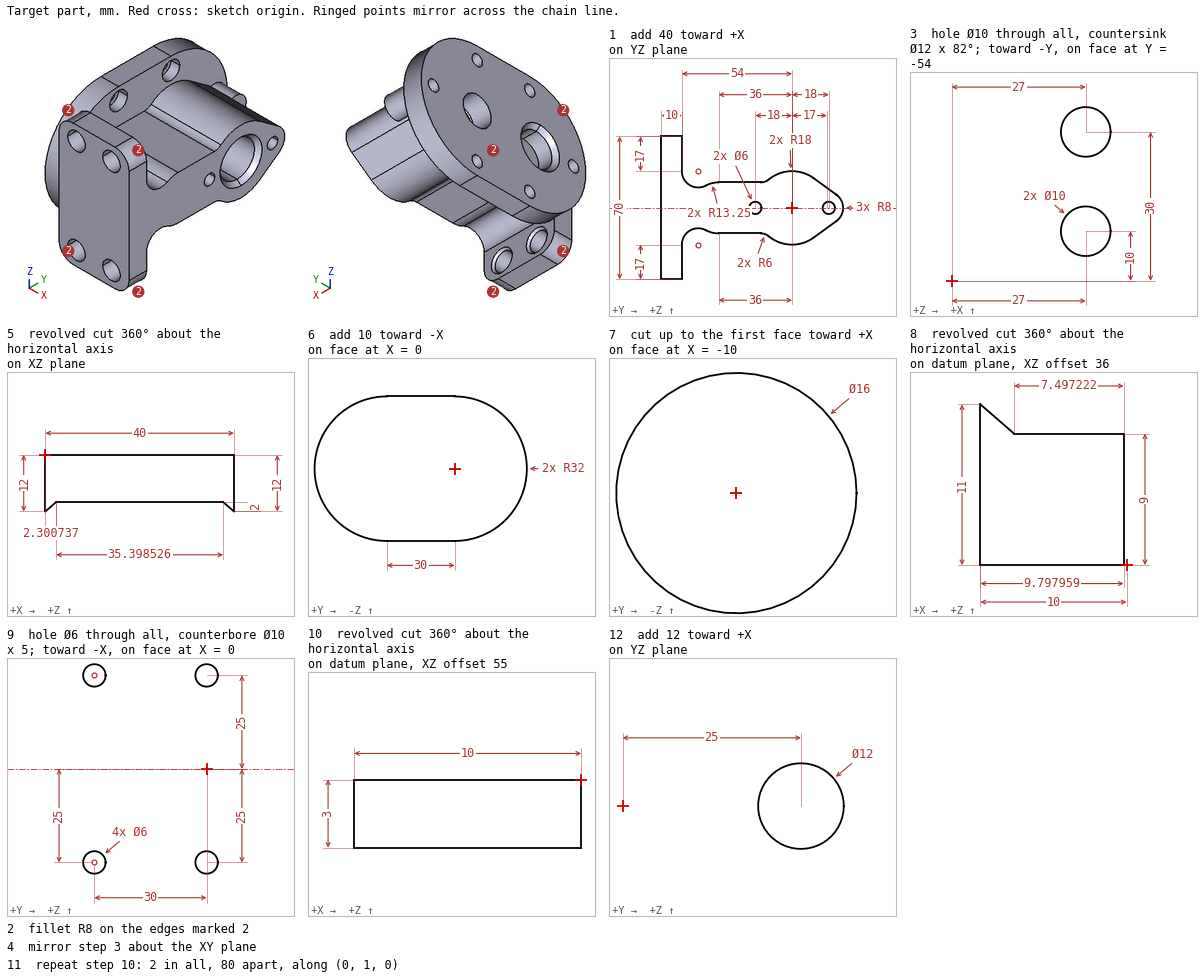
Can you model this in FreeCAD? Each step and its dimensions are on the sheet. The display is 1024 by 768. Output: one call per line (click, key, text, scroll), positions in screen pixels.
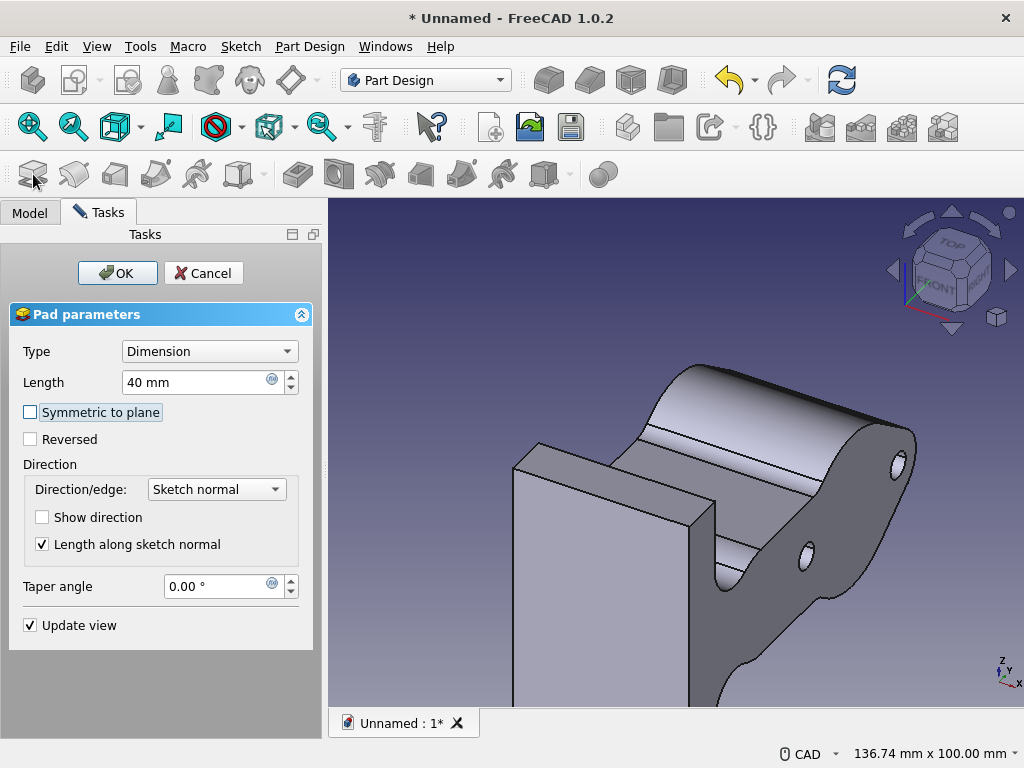
click(118, 273)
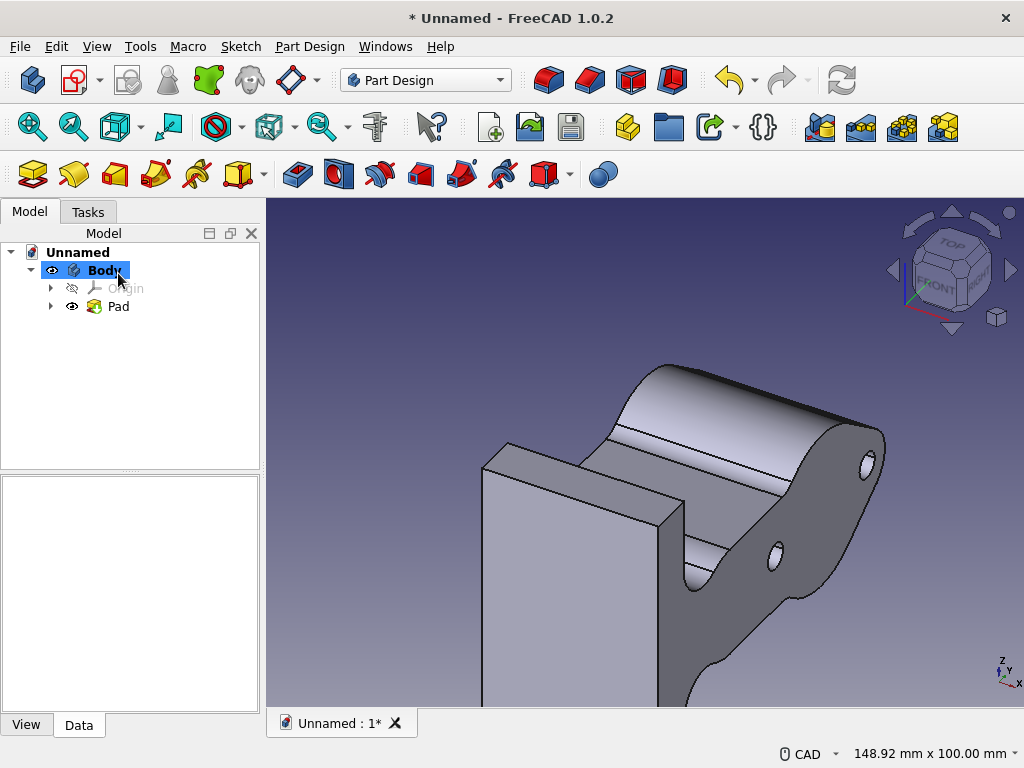
click(33, 128)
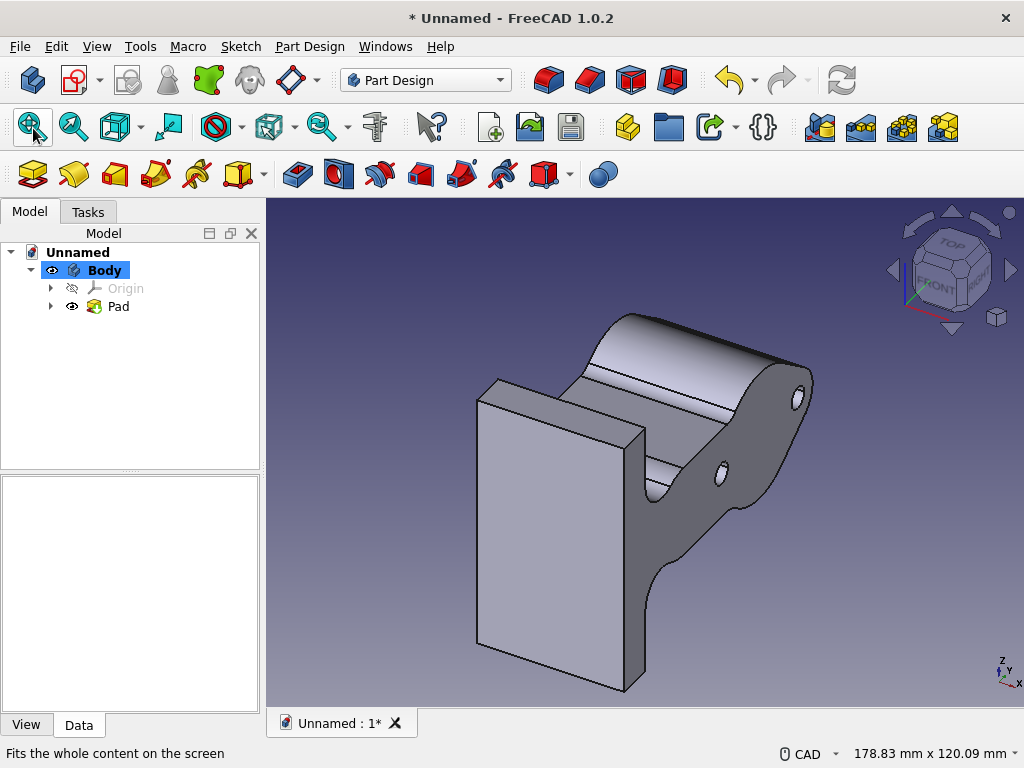
click(635, 437)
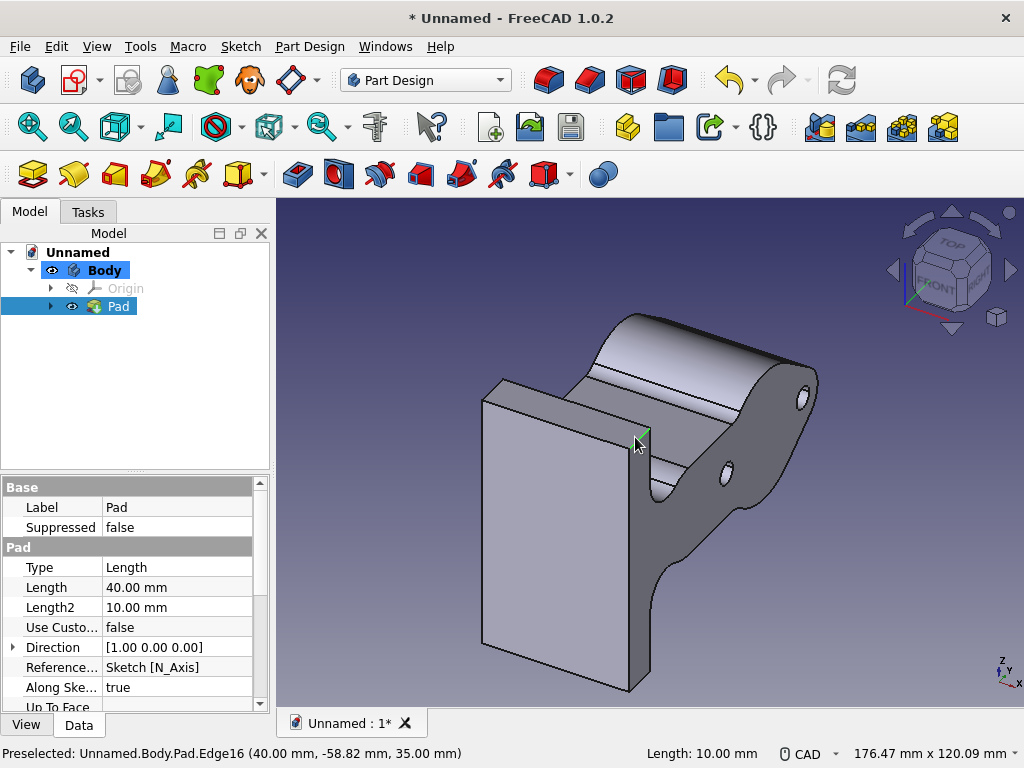
key(0)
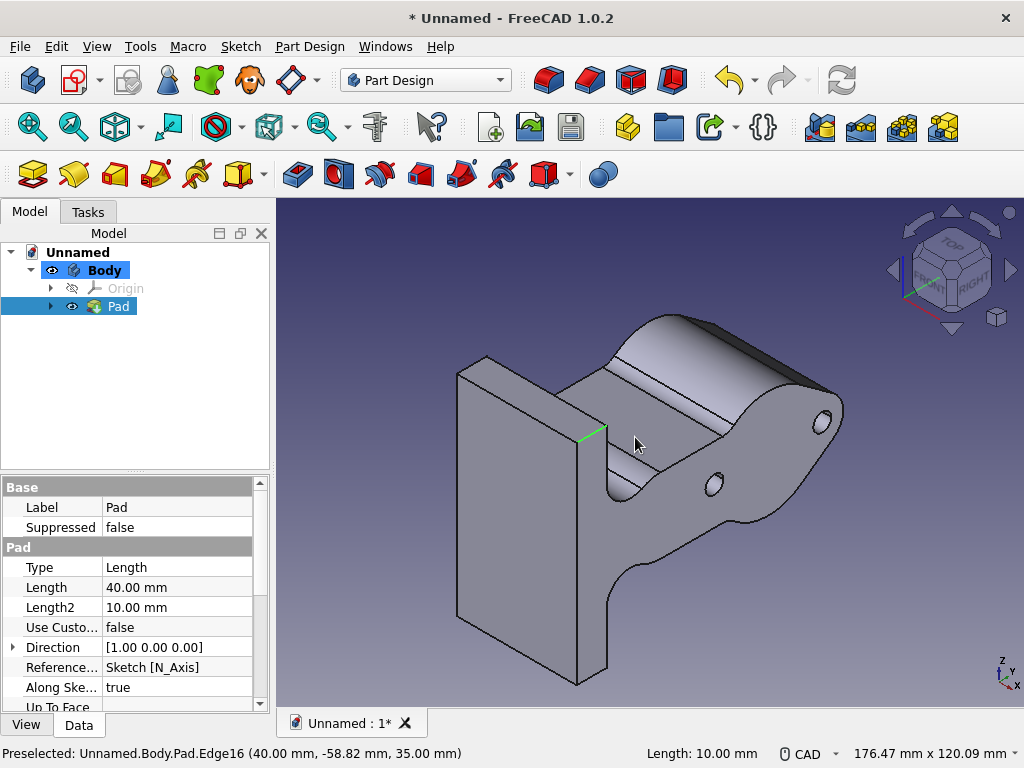
key(2)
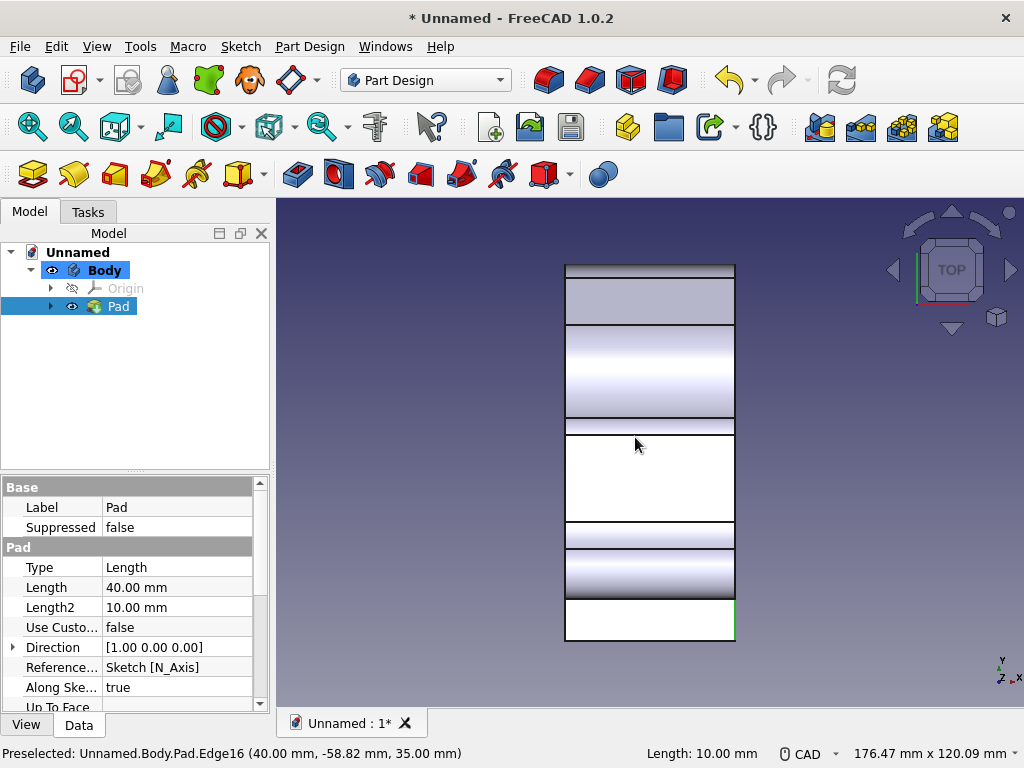
click(565, 619, ctrl)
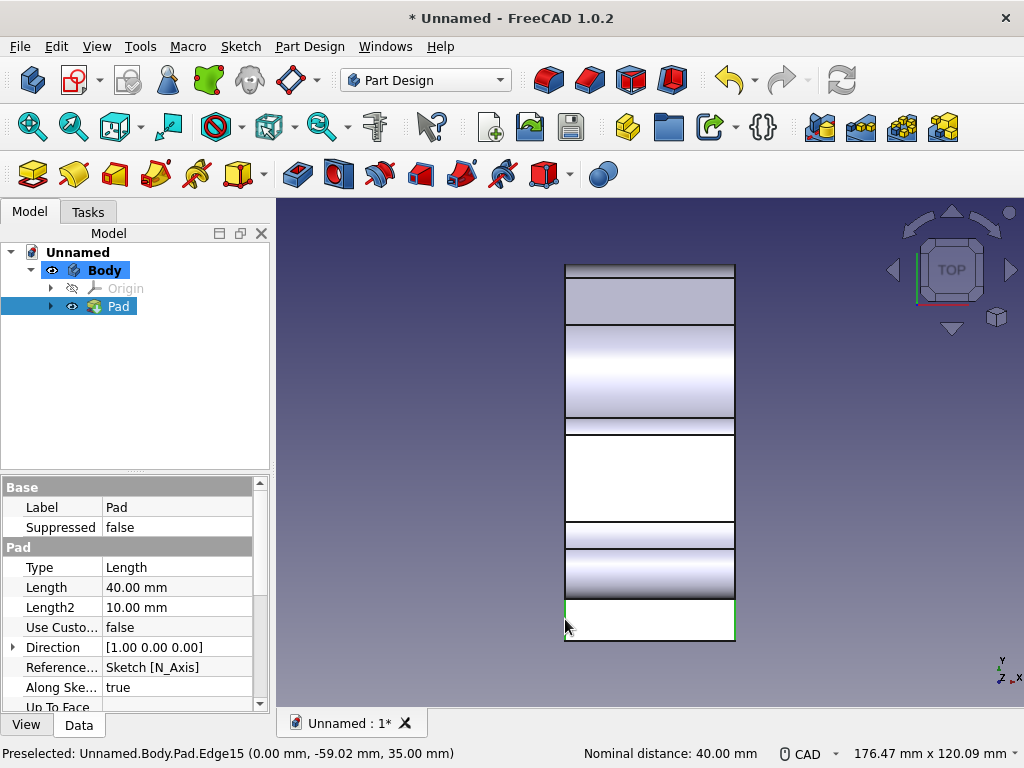
key(1)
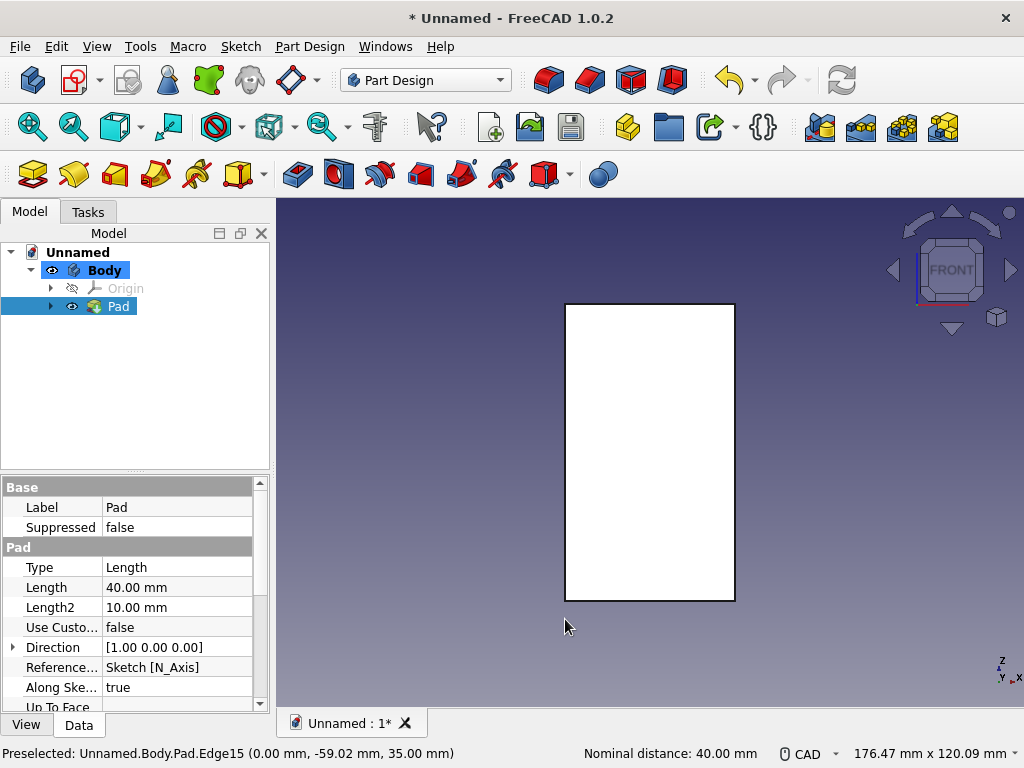
key(3)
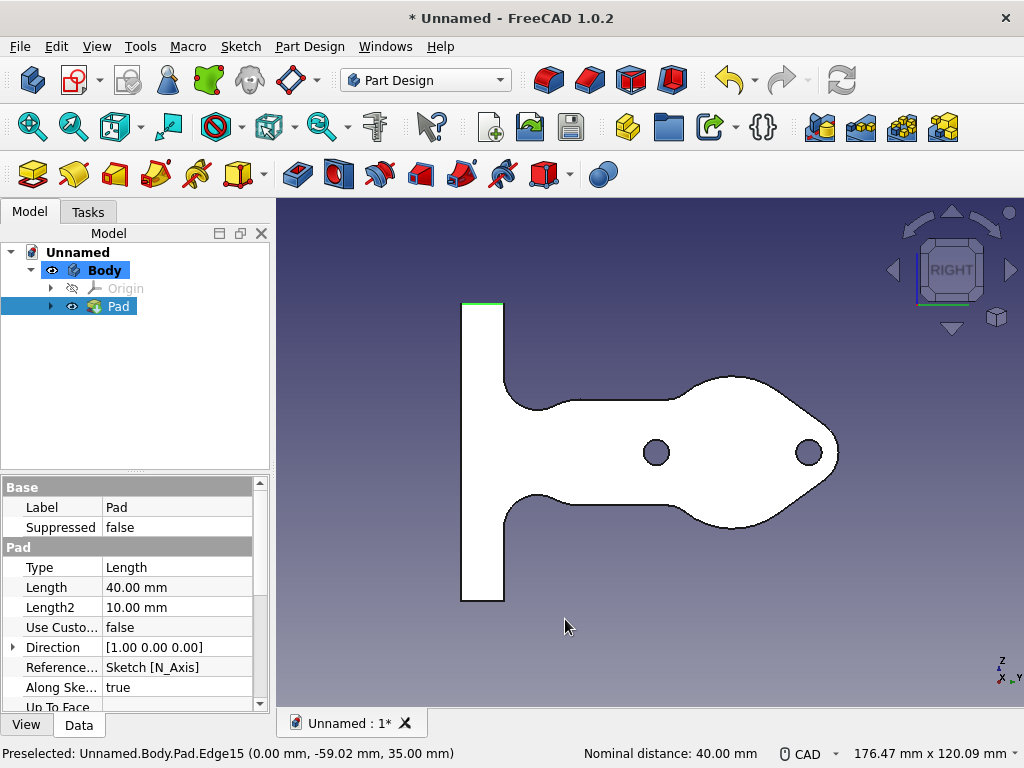
click(483, 600, ctrl)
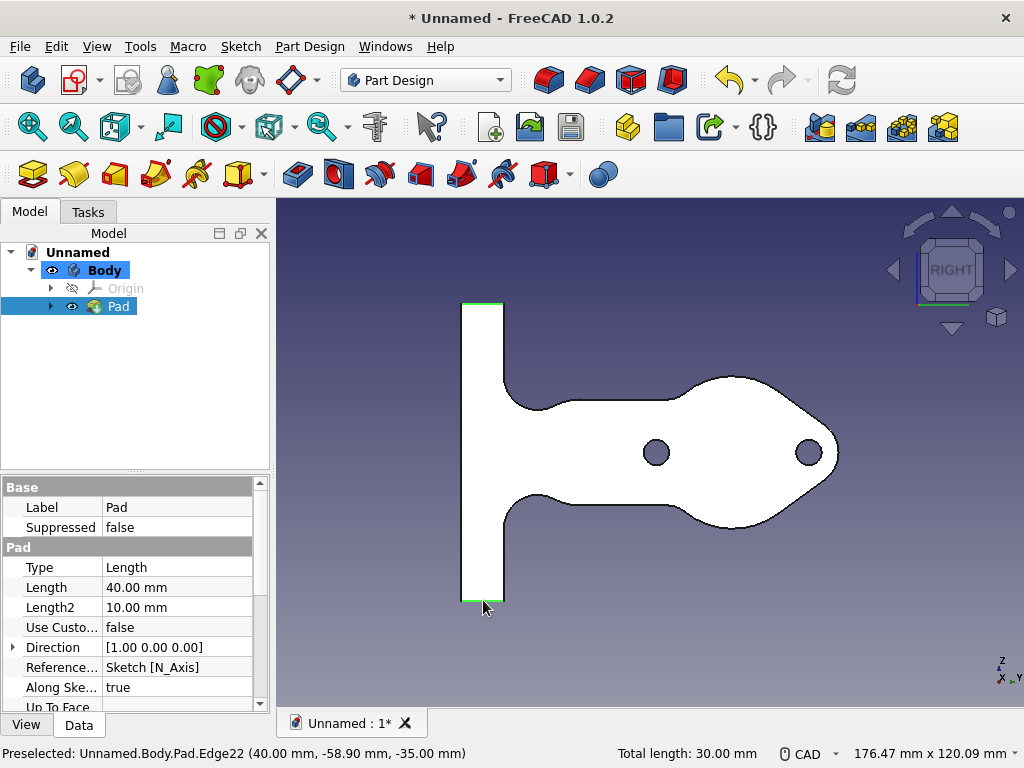
key(5)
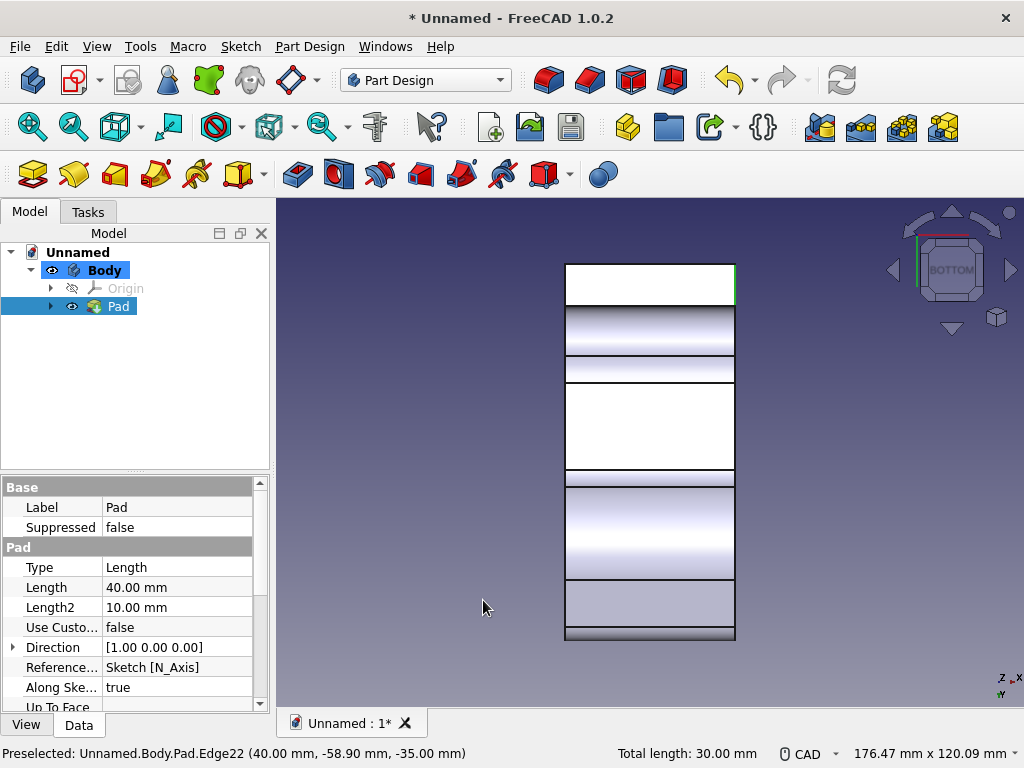
click(565, 284, ctrl)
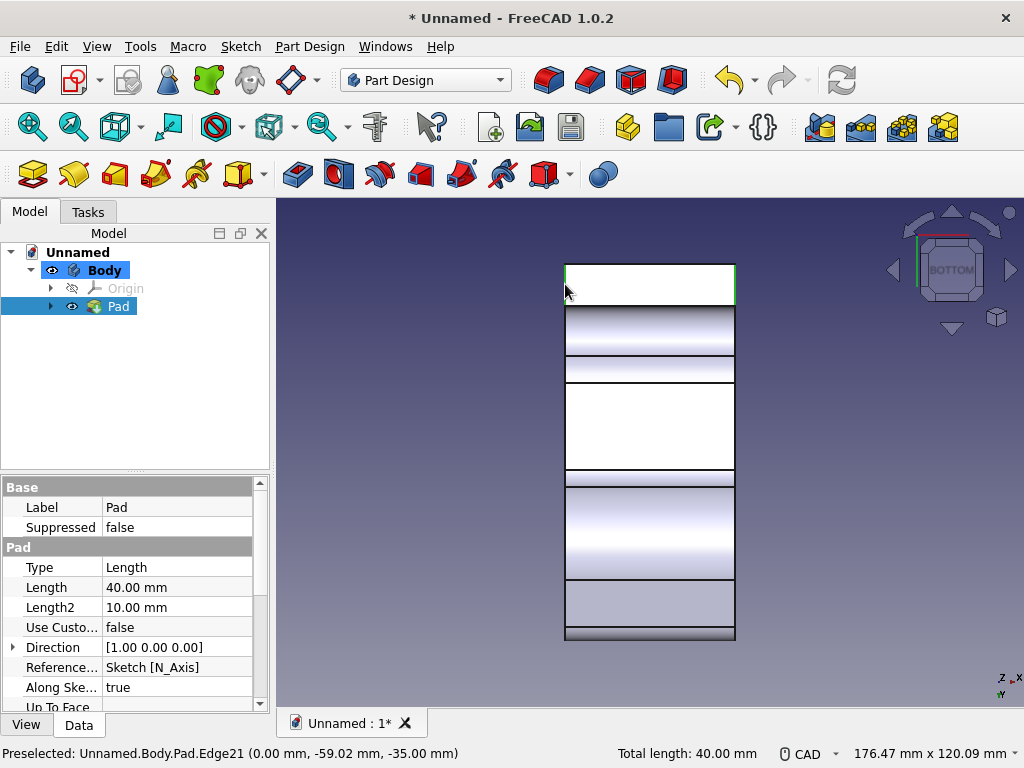
click(549, 80)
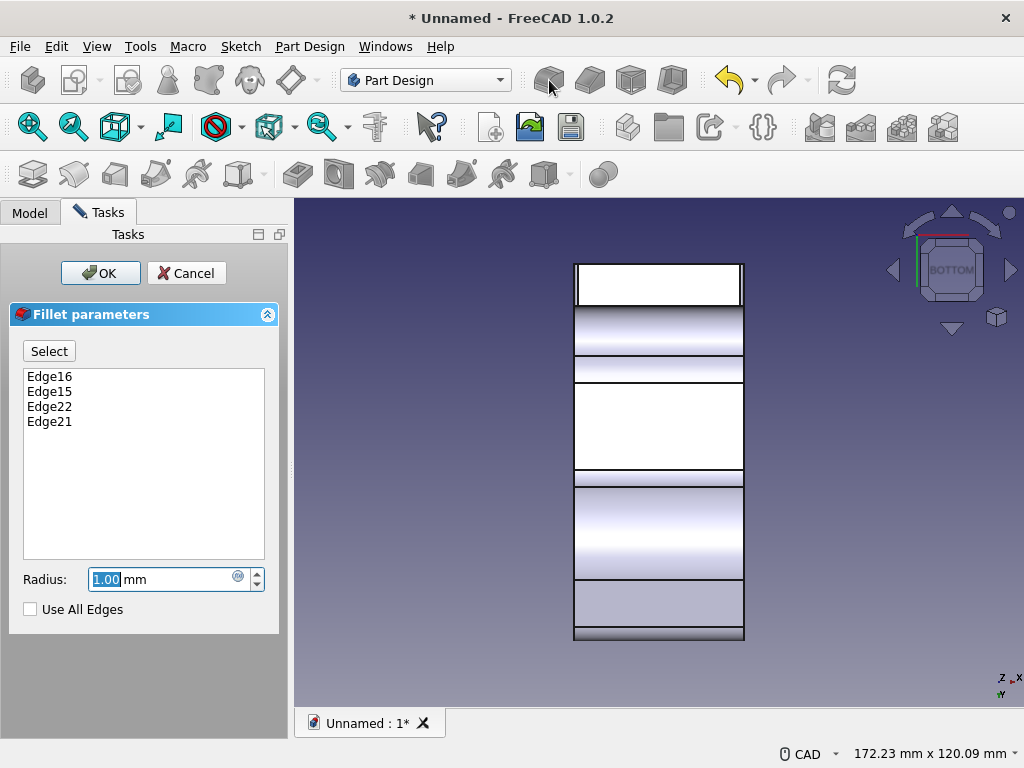
text(8)
key(Tab)